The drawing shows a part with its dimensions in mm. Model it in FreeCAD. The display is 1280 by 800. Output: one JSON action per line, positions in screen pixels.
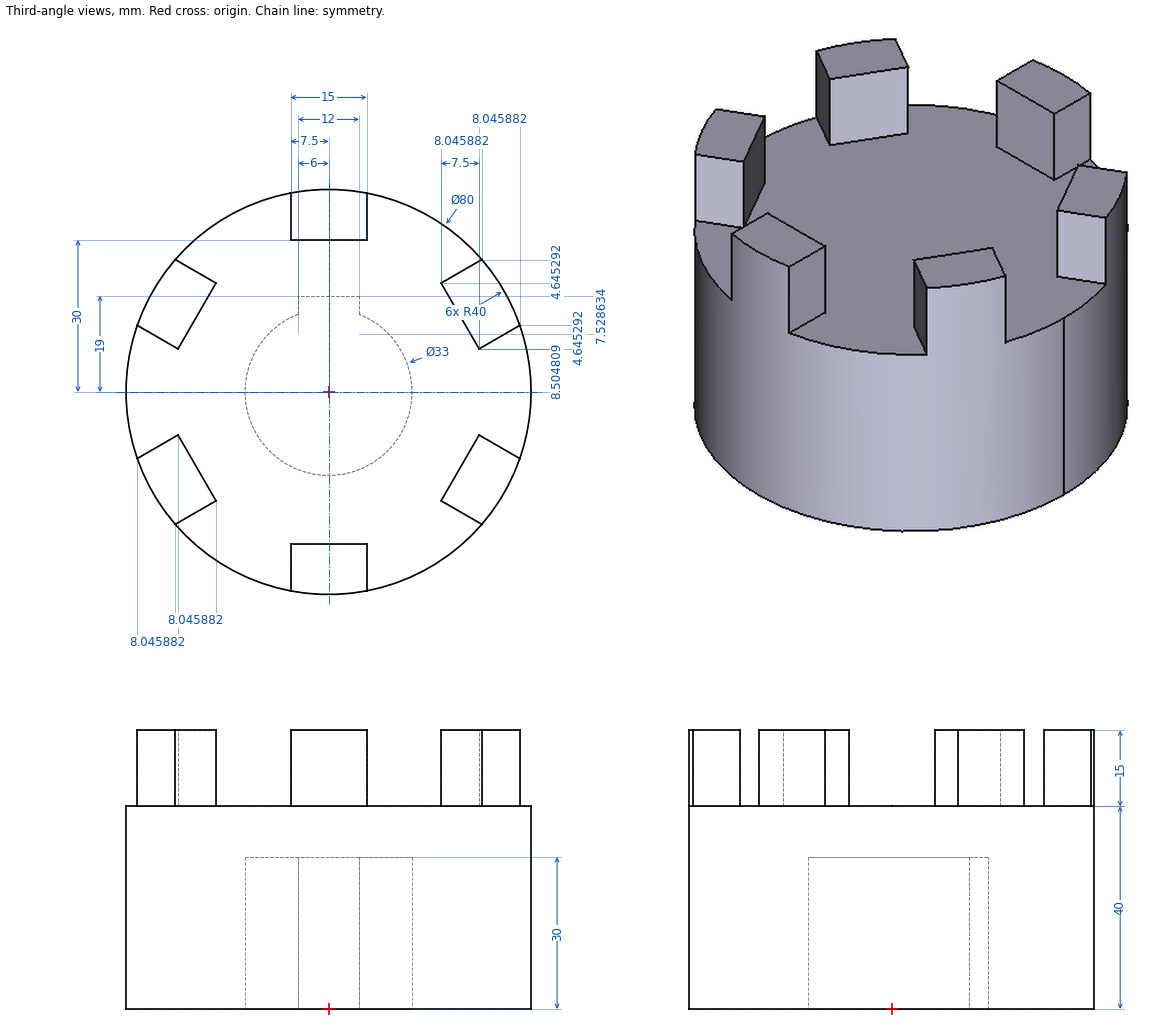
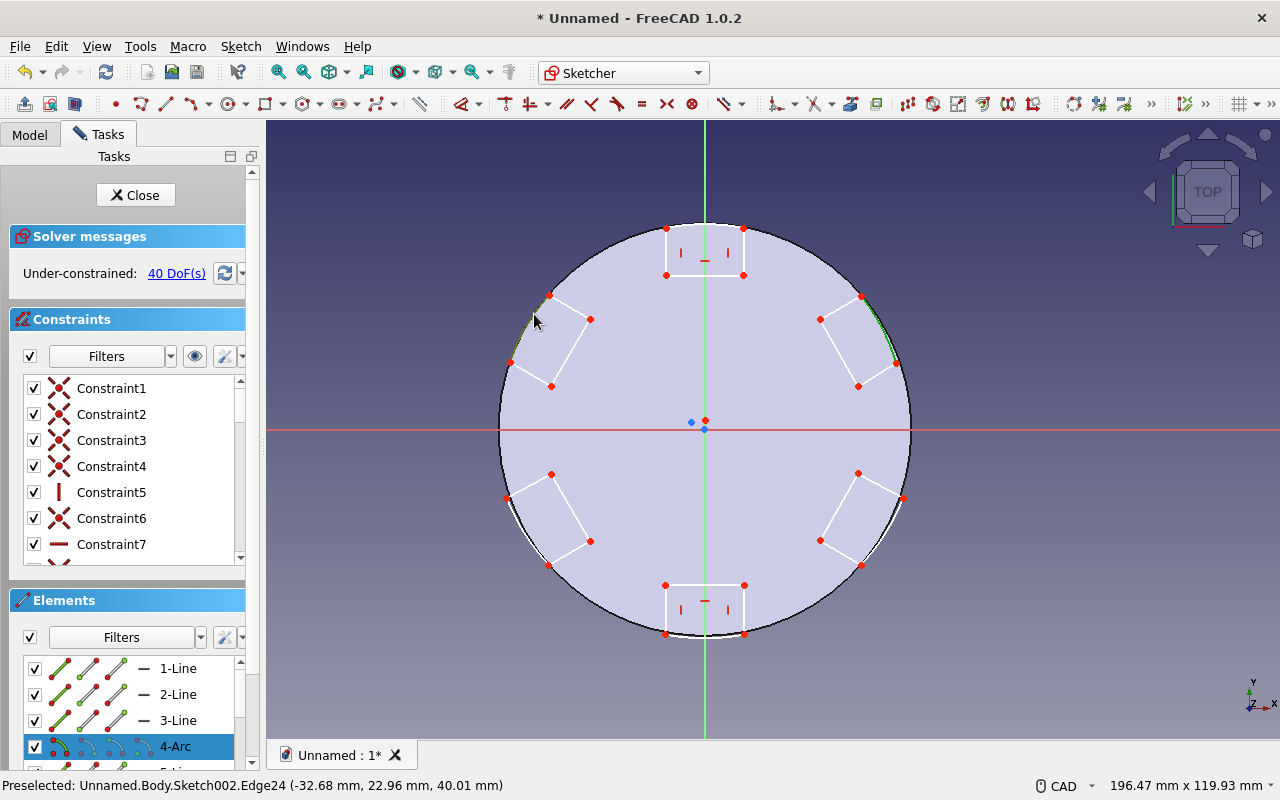
{"action": "key", "text": "c"}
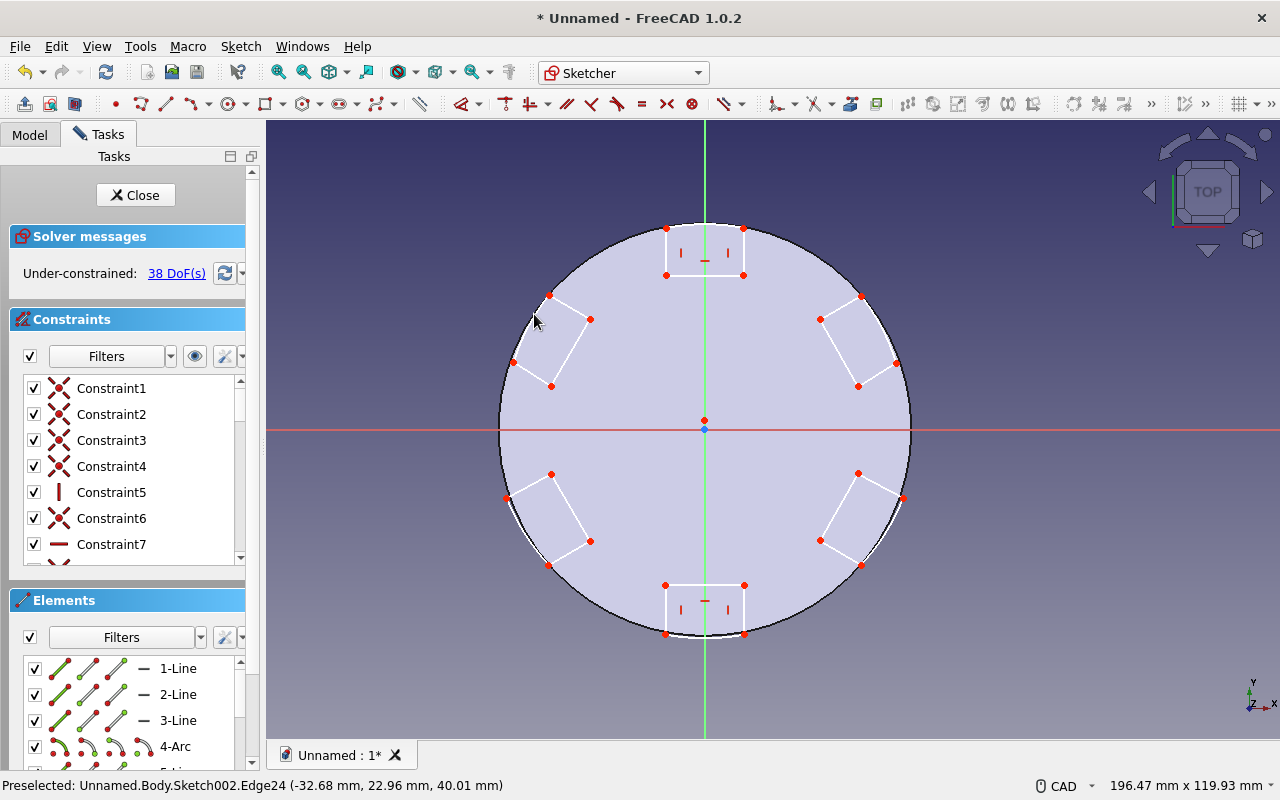
{"action": "left_click_drag", "start_coordinate": [695, 410], "coordinate": [715, 439]}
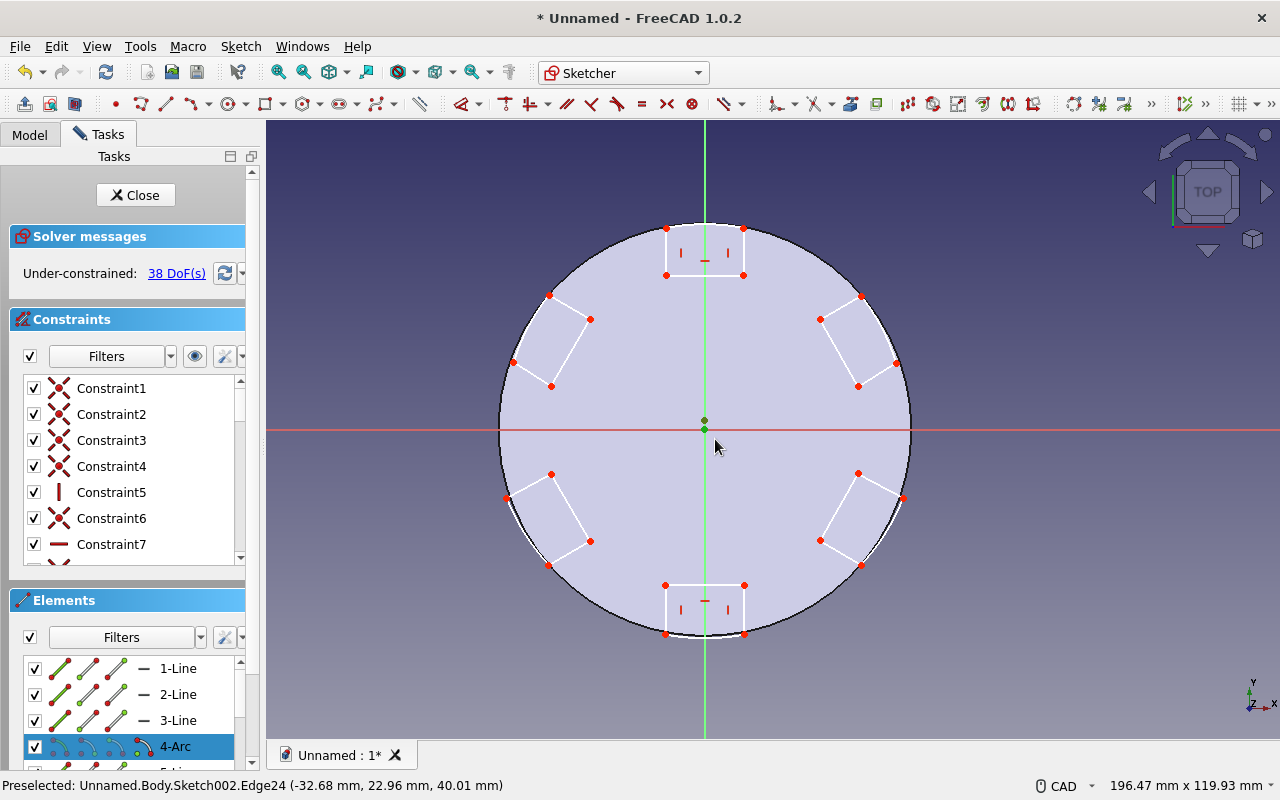
{"action": "left_click", "coordinate": [505, 104]}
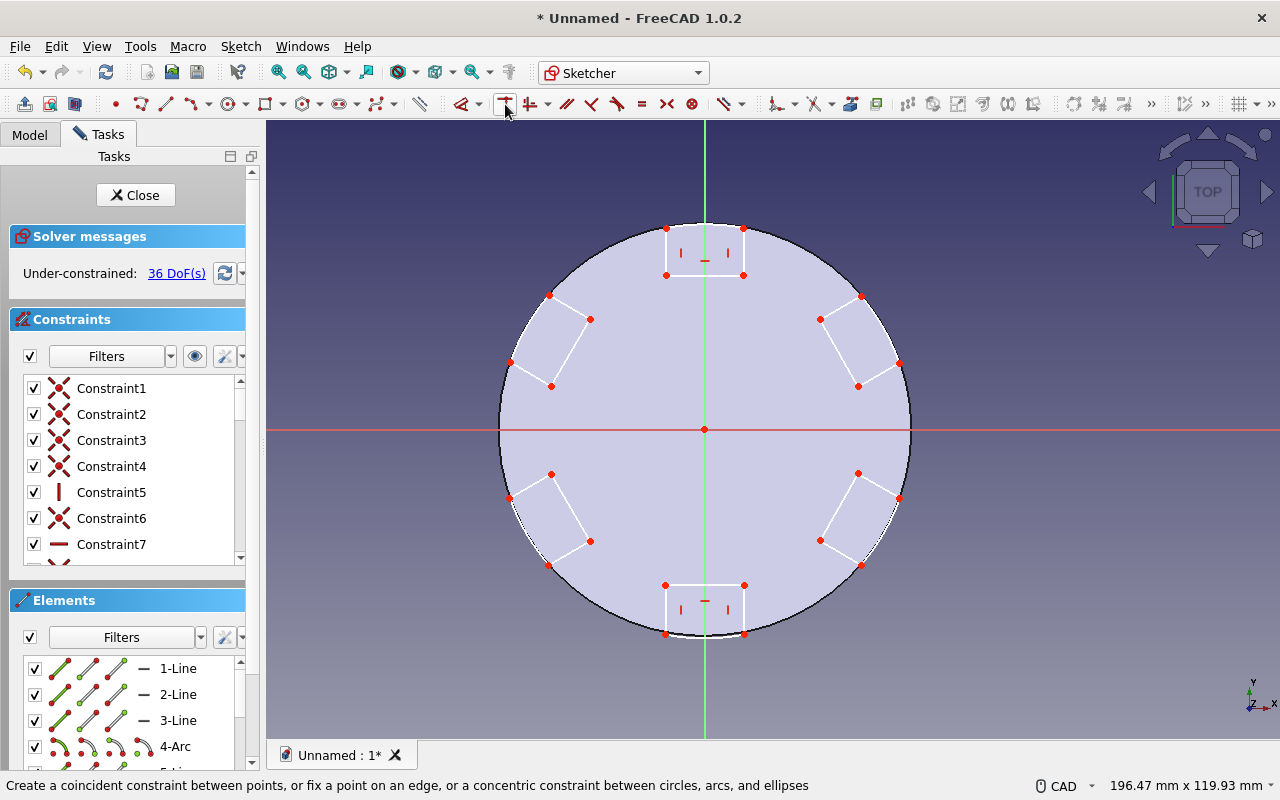
{"action": "left_click", "coordinate": [890, 341]}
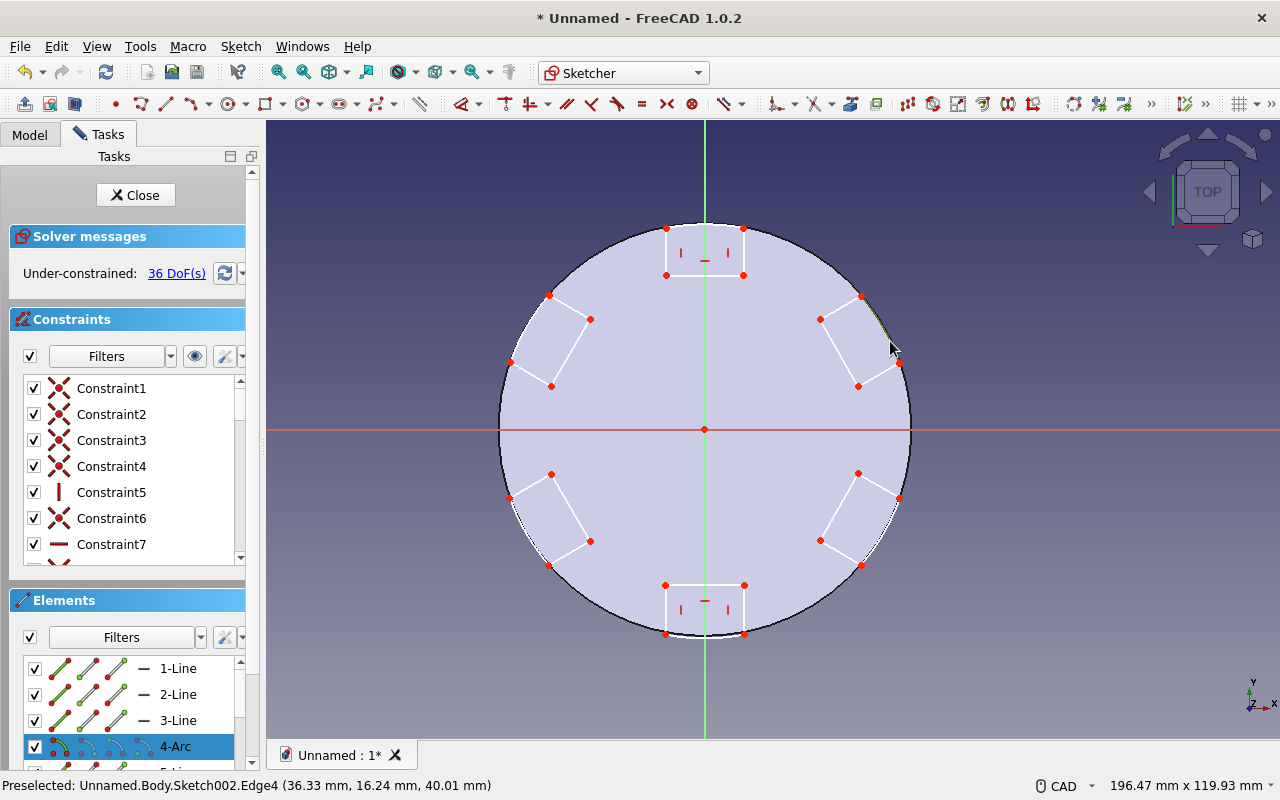
{"action": "left_click", "coordinate": [721, 225]}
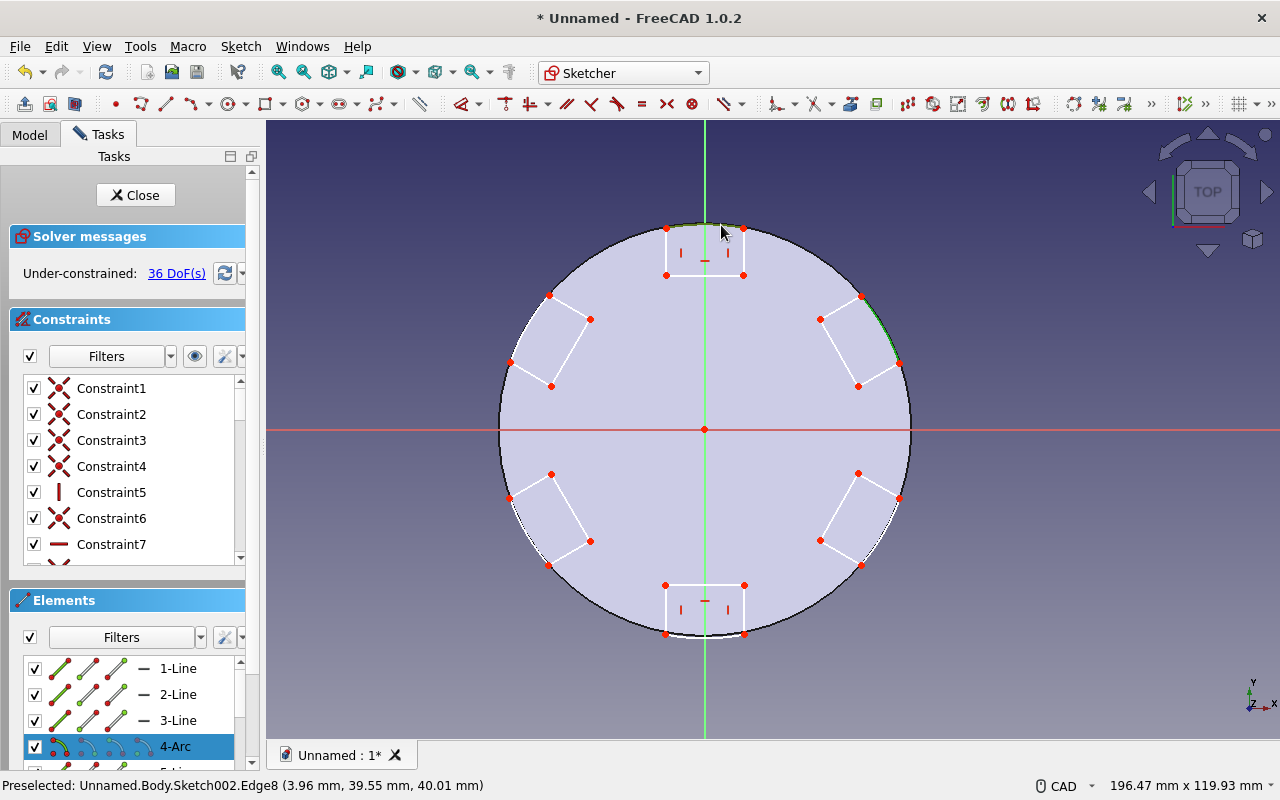
{"action": "left_click", "coordinate": [875, 547]}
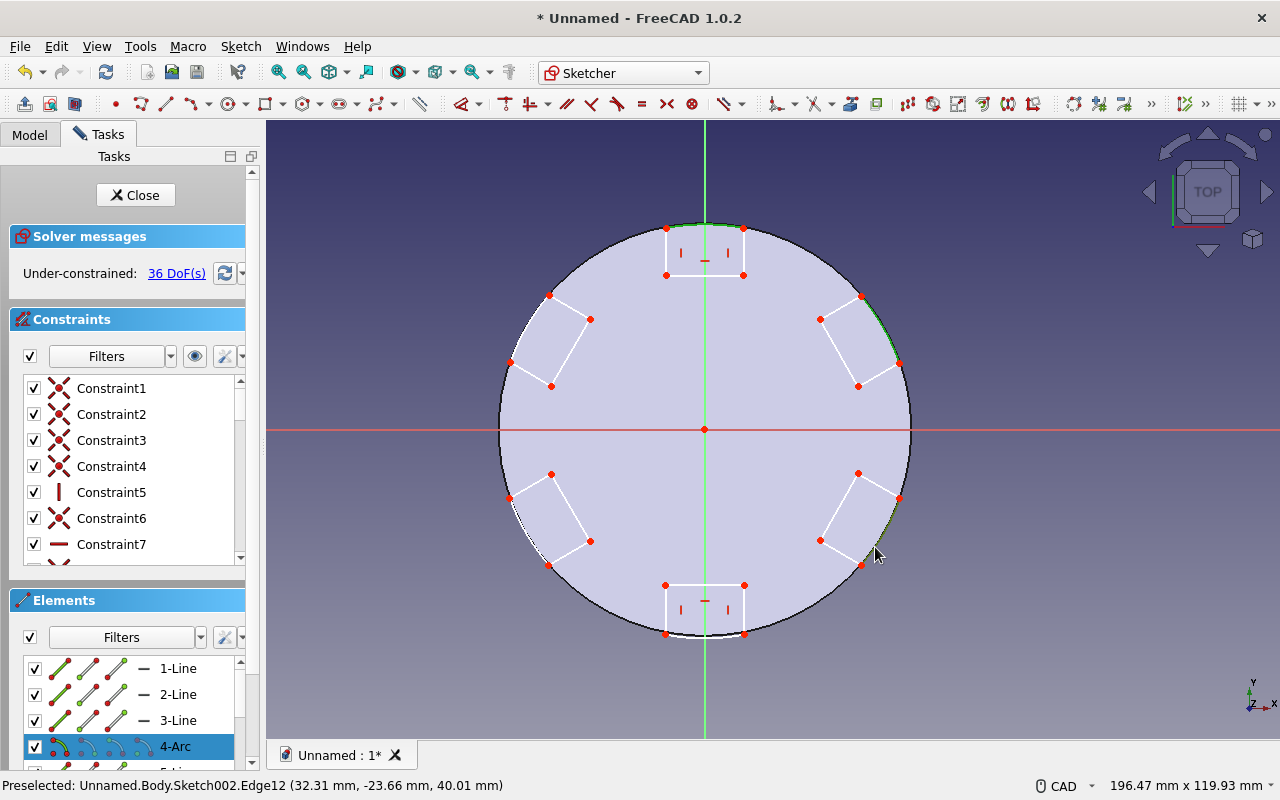
{"action": "left_click", "coordinate": [689, 638]}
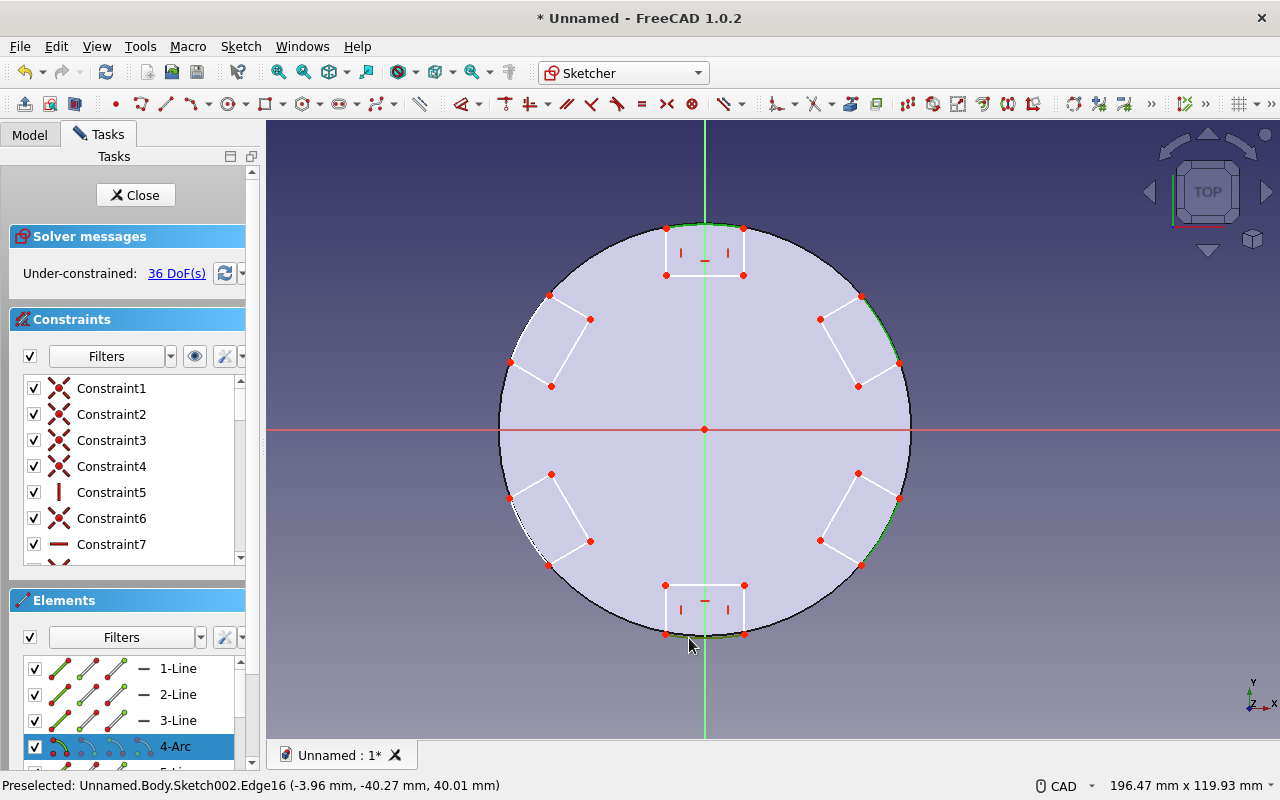
{"action": "left_click", "coordinate": [519, 520]}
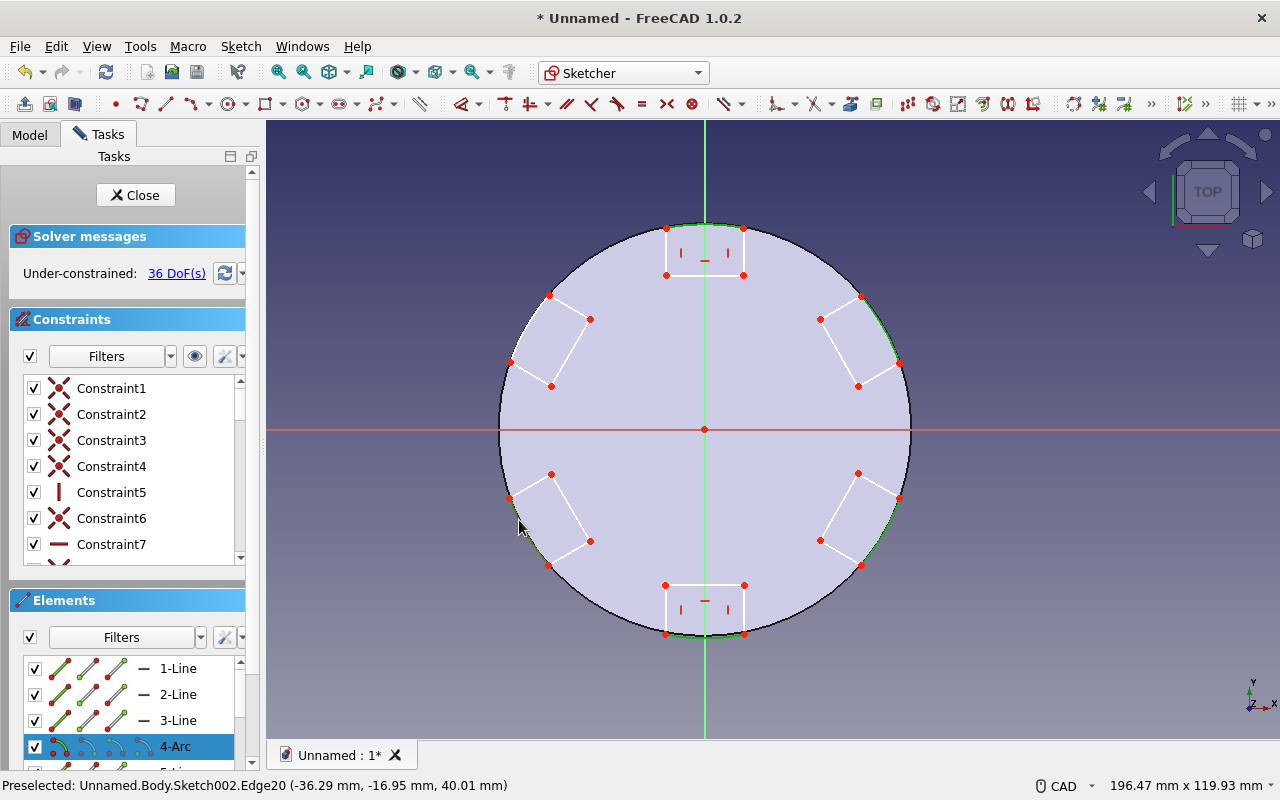
{"action": "left_click", "coordinate": [535, 314]}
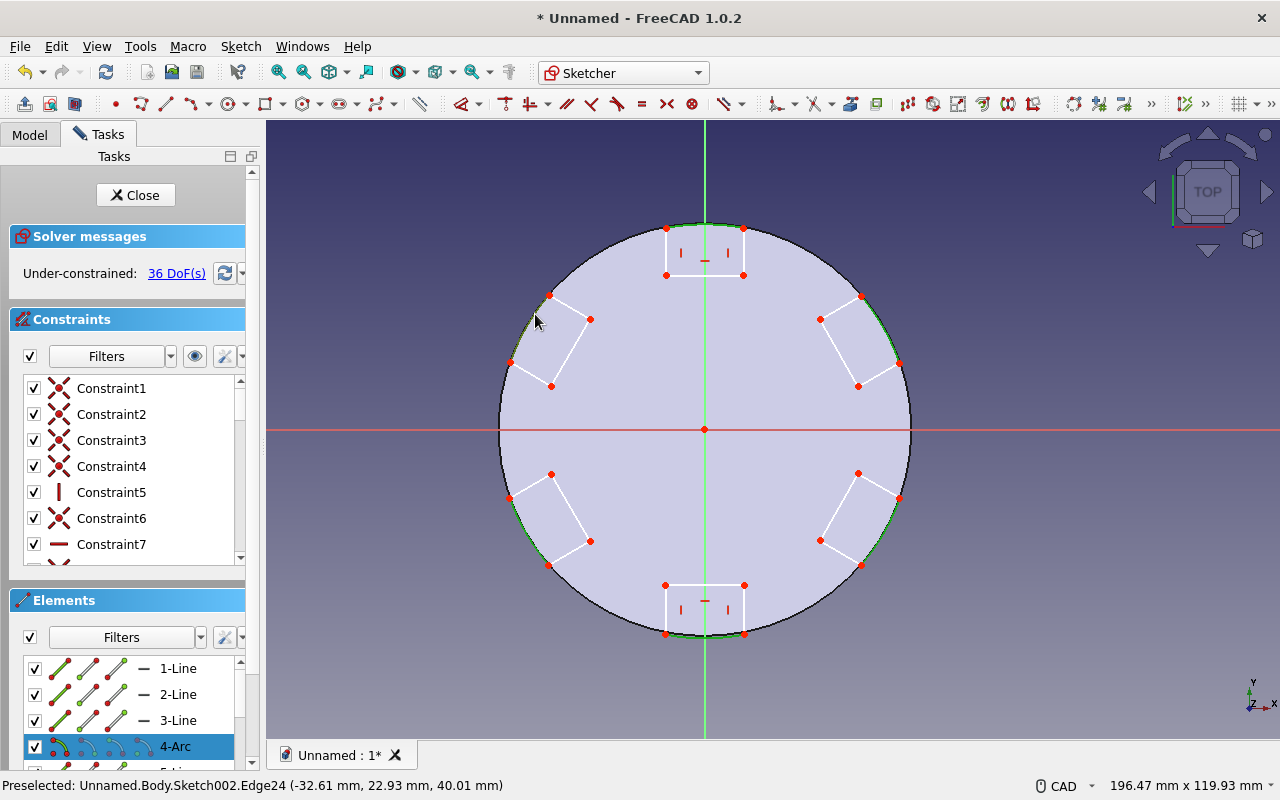
{"action": "key", "text": "e"}